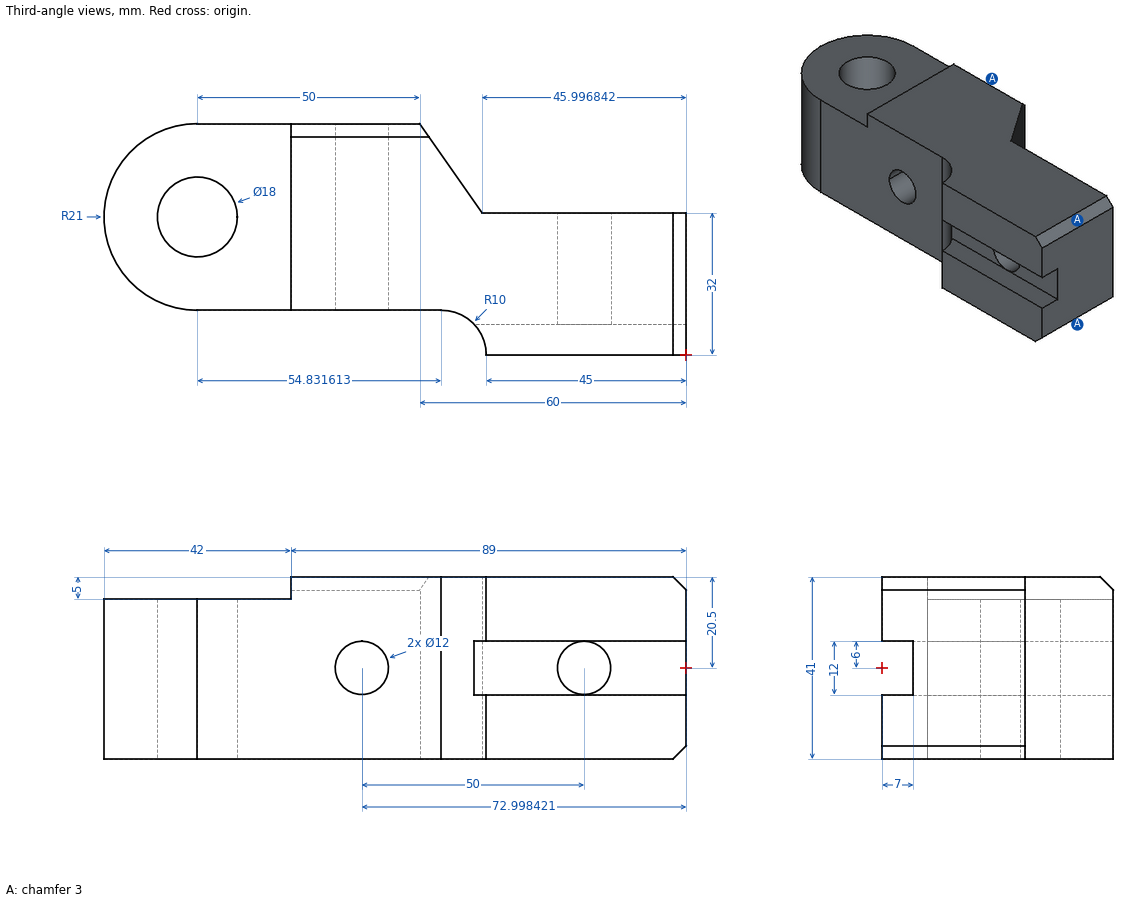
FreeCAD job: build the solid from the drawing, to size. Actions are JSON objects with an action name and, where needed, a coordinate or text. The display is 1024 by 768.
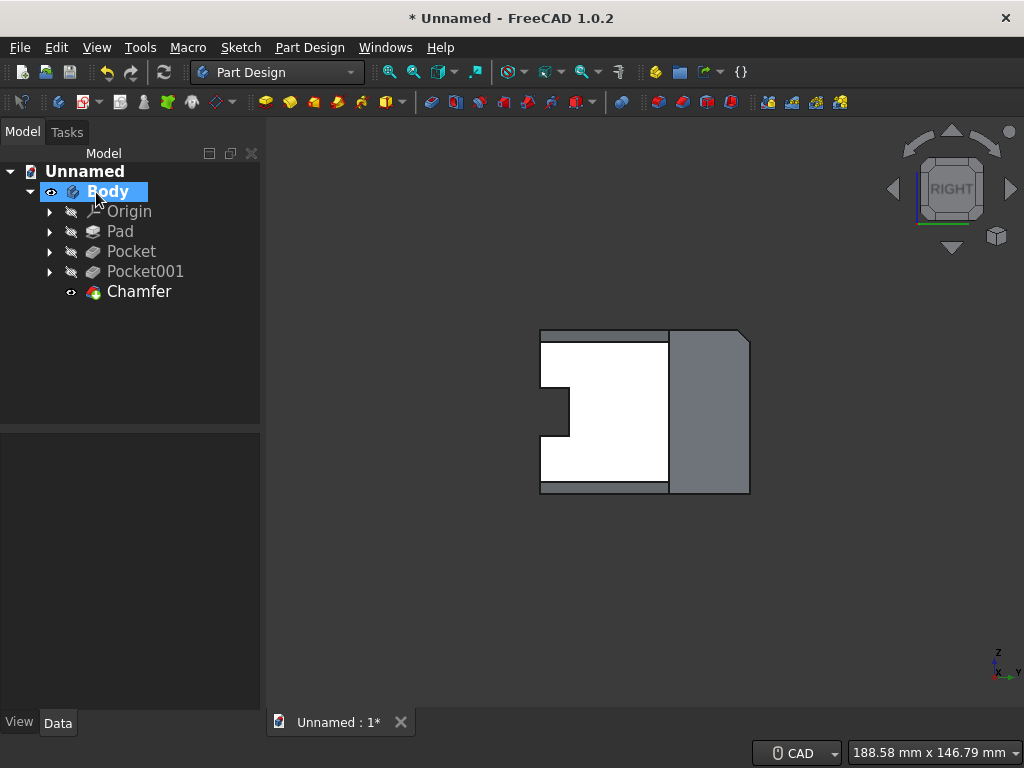
{"action": "key", "text": "0"}